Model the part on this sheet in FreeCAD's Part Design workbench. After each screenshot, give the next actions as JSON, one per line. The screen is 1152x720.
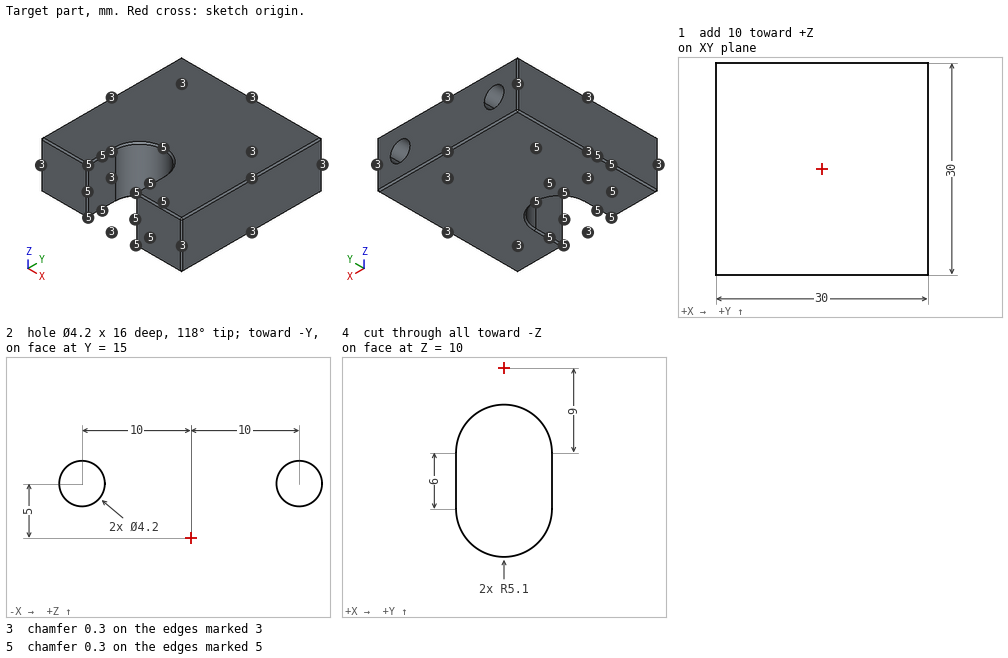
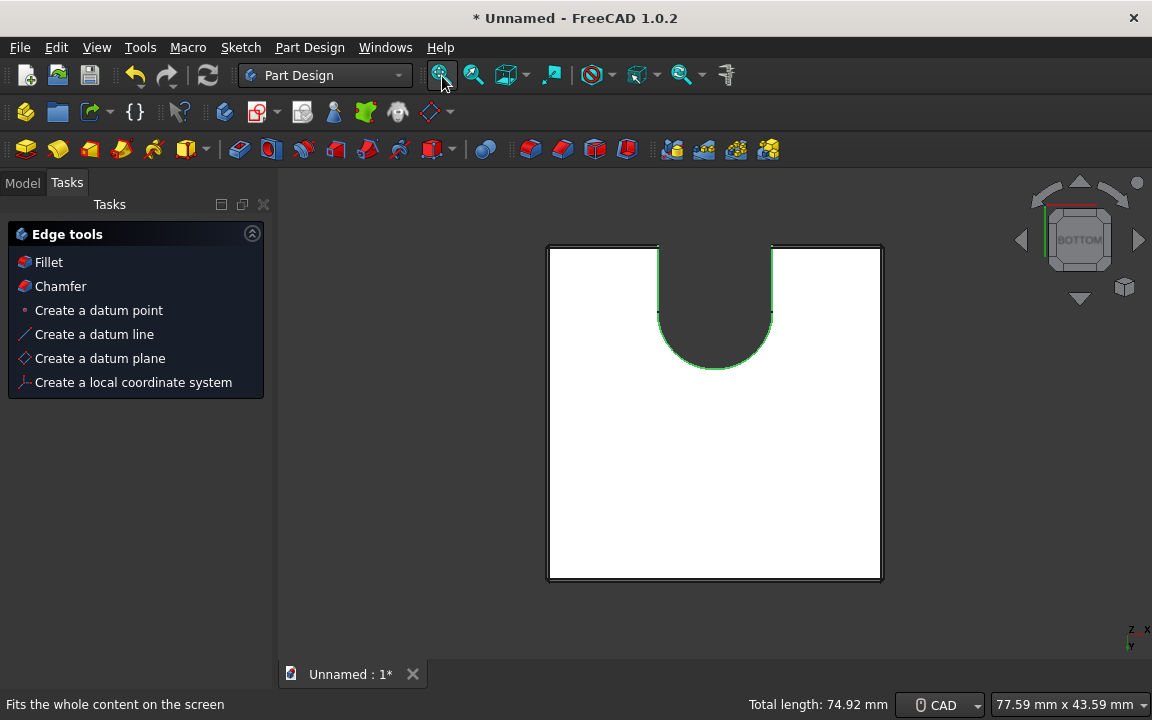
{"action": "key", "text": "4"}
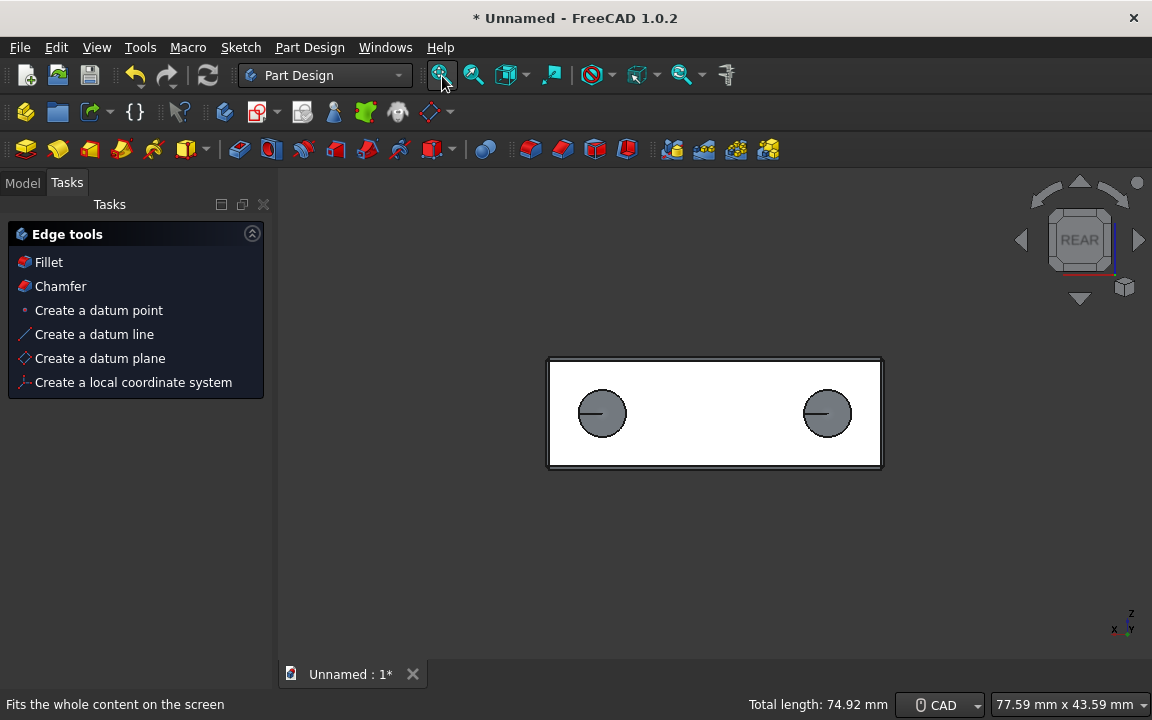
{"action": "left_click", "coordinate": [442, 76]}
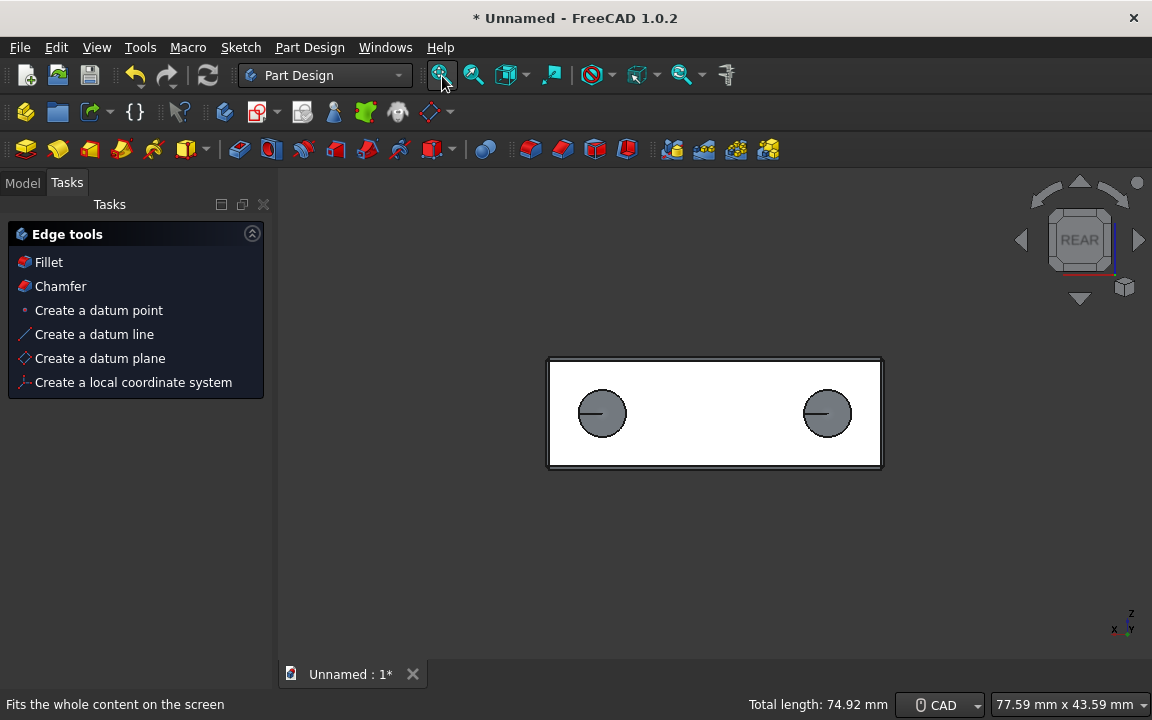
{"action": "scroll", "coordinate": [772, 358], "scroll_direction": "up", "scroll_amount": 11}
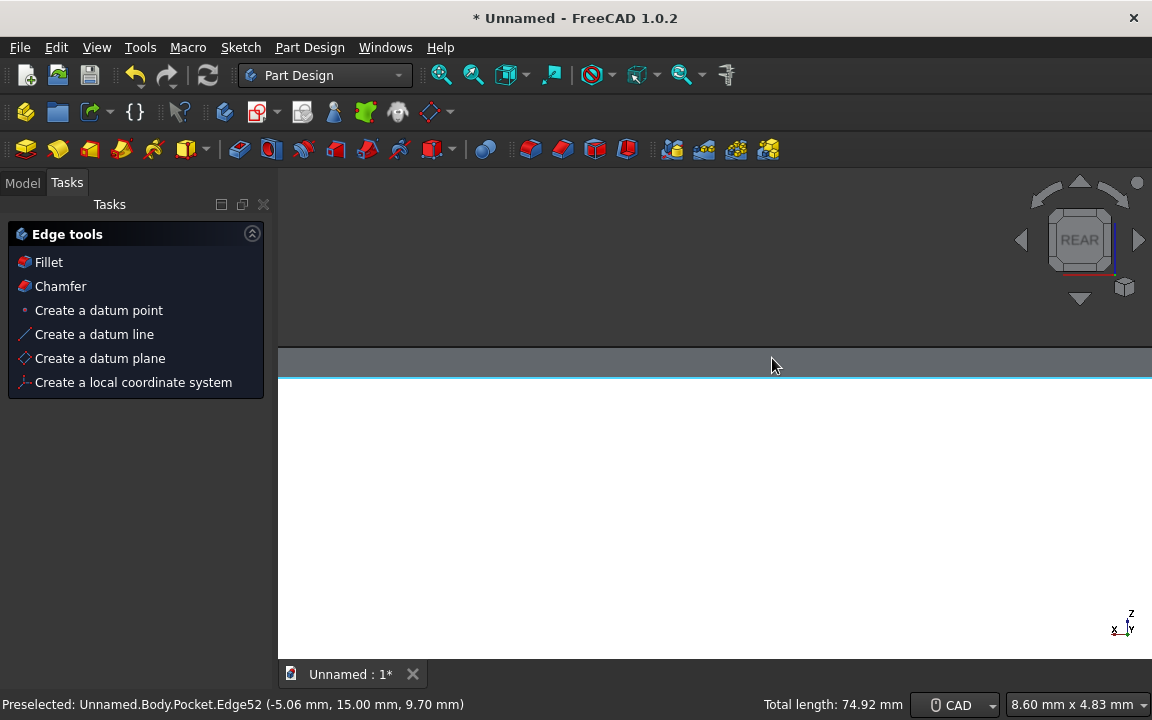
{"action": "left_click", "coordinate": [442, 76]}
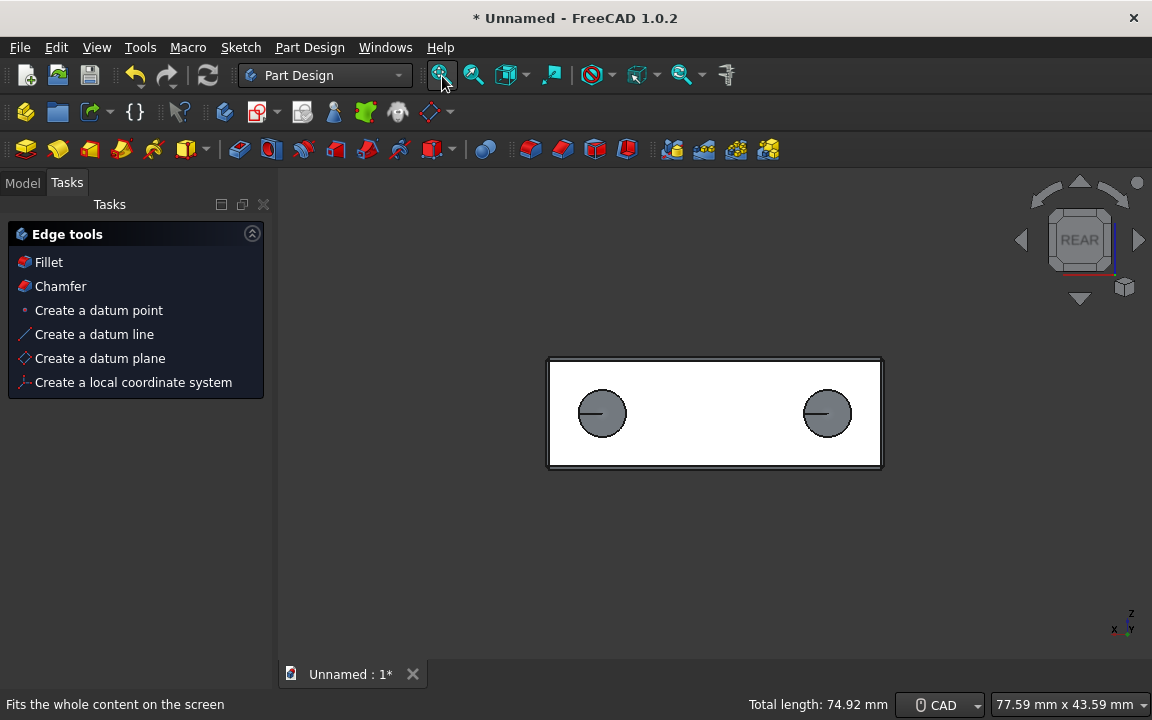
{"action": "key", "text": "6"}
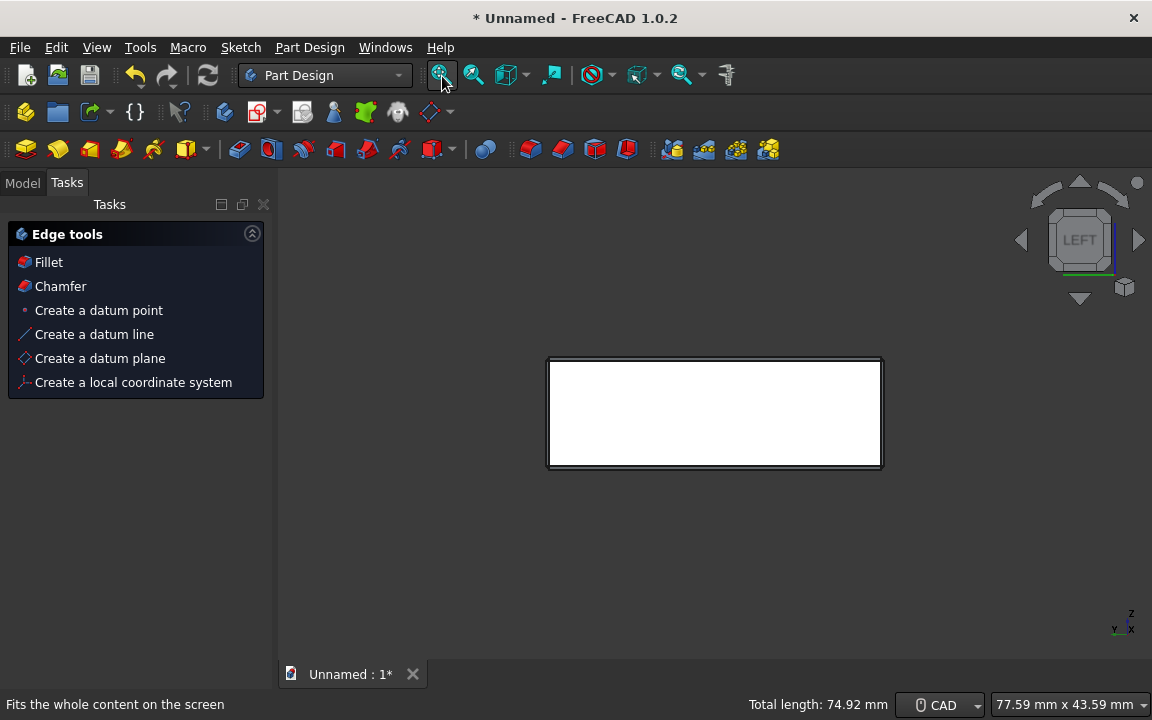
{"action": "left_click", "coordinate": [442, 76]}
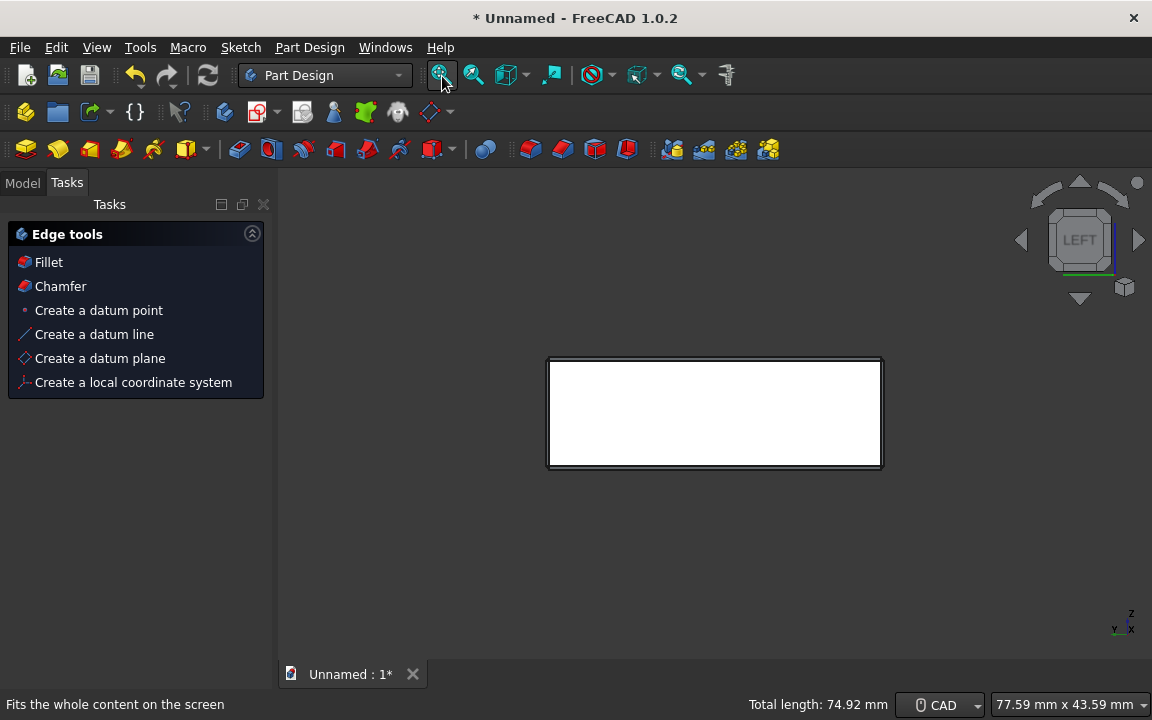
{"action": "scroll", "coordinate": [882, 358], "scroll_direction": "up", "scroll_amount": 11}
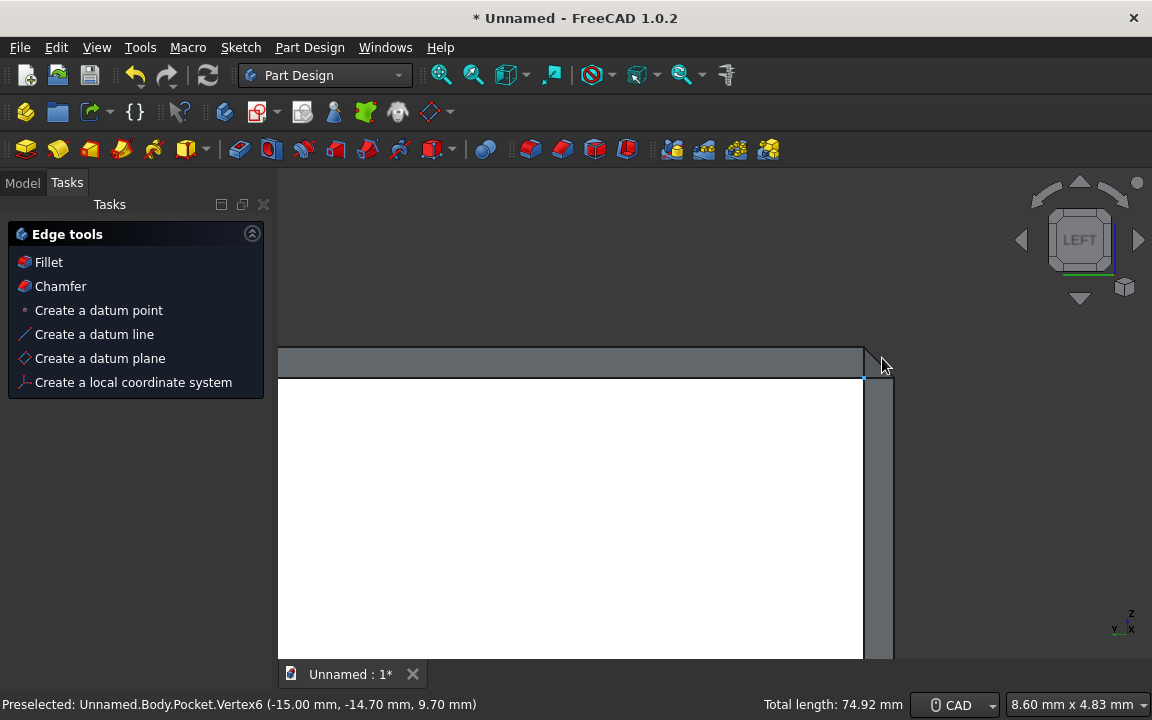
{"action": "left_click", "coordinate": [442, 76]}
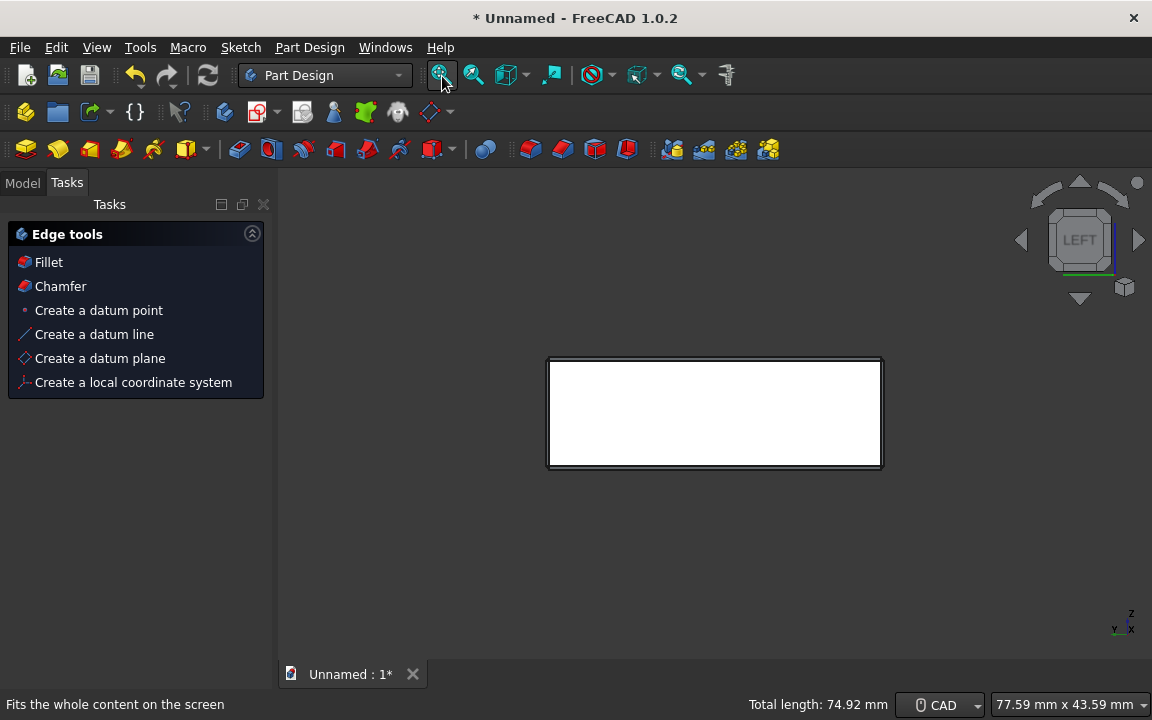
{"action": "key", "text": "v 3"}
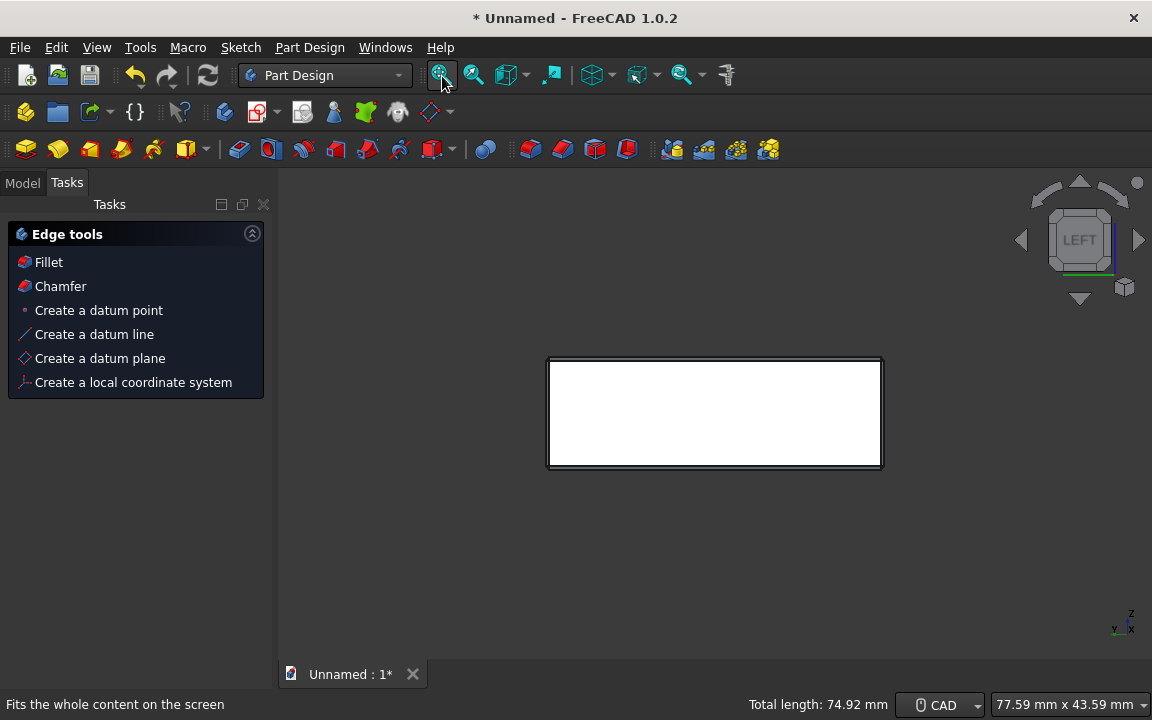
{"action": "key", "text": "0"}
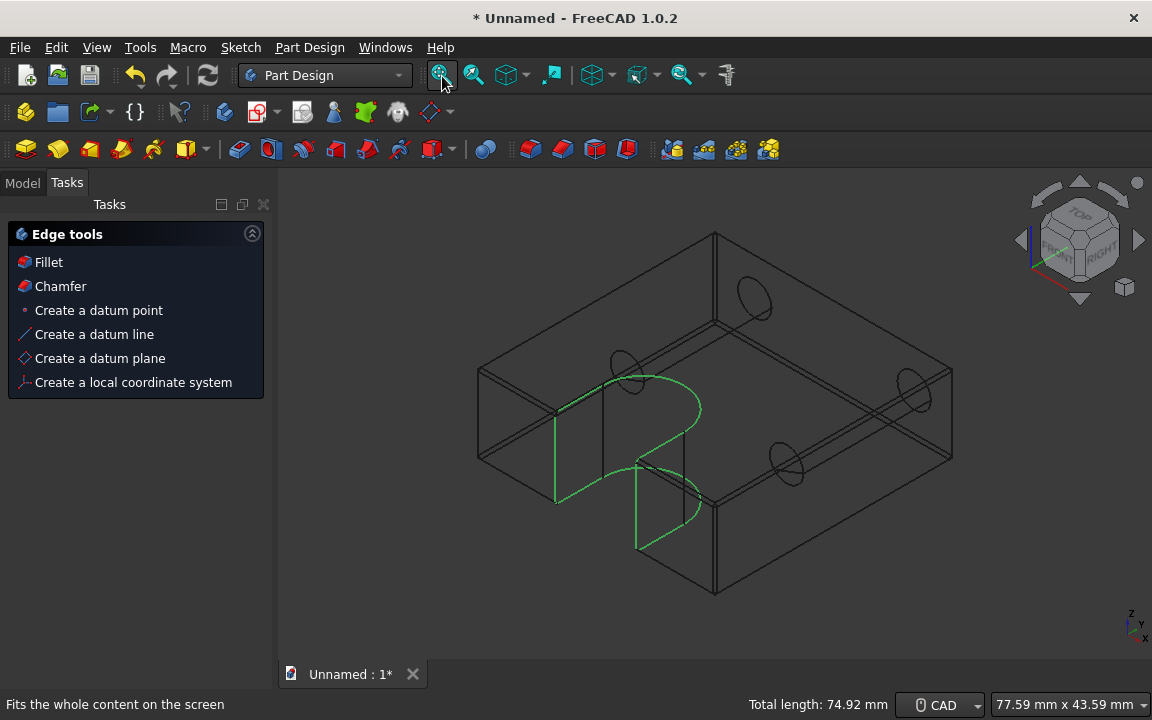
{"action": "scroll", "coordinate": [556, 413], "scroll_direction": "up", "scroll_amount": 11}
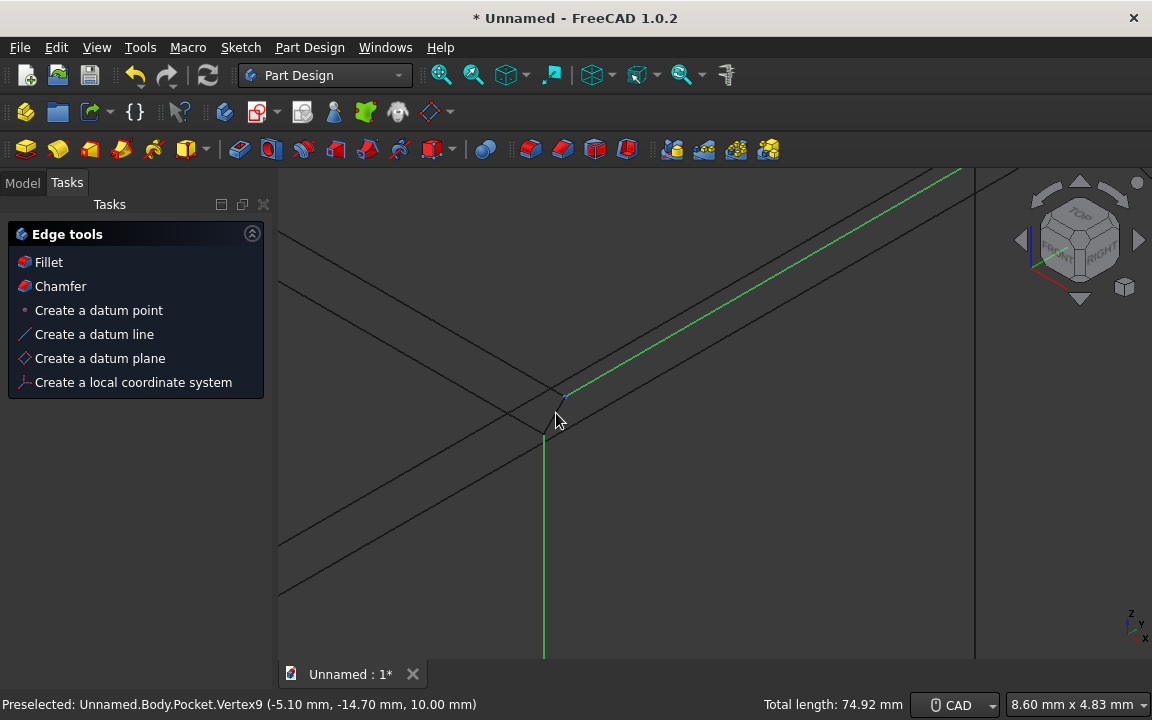
{"action": "left_click", "coordinate": [554, 415], "text": "ctrl"}